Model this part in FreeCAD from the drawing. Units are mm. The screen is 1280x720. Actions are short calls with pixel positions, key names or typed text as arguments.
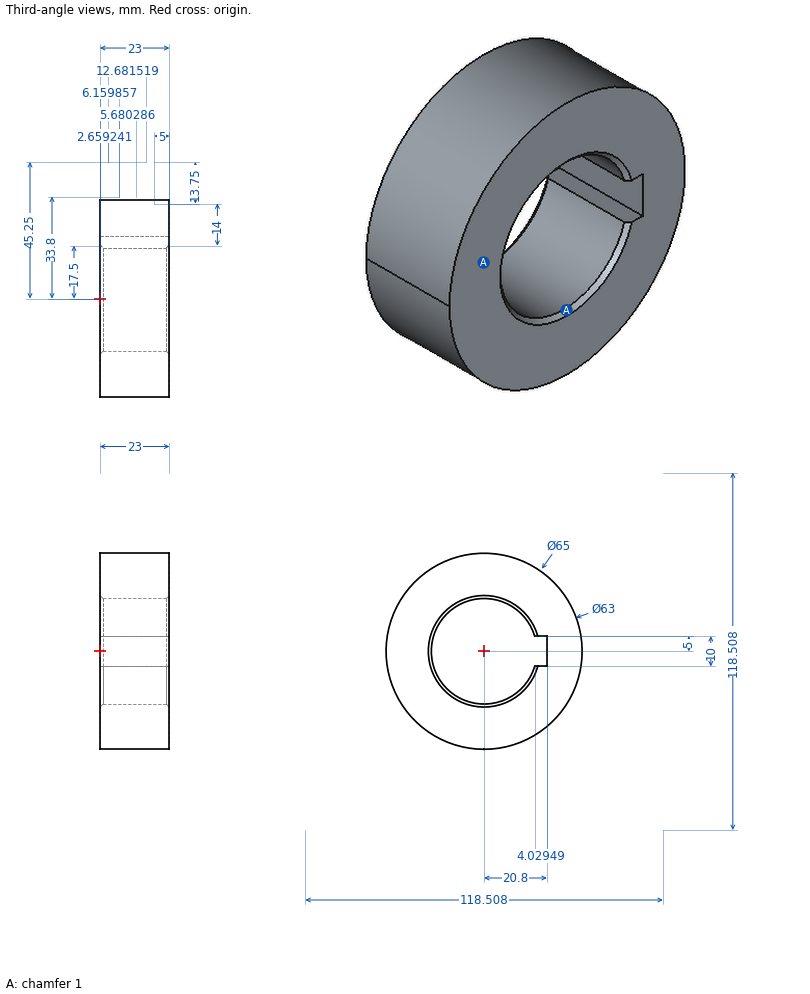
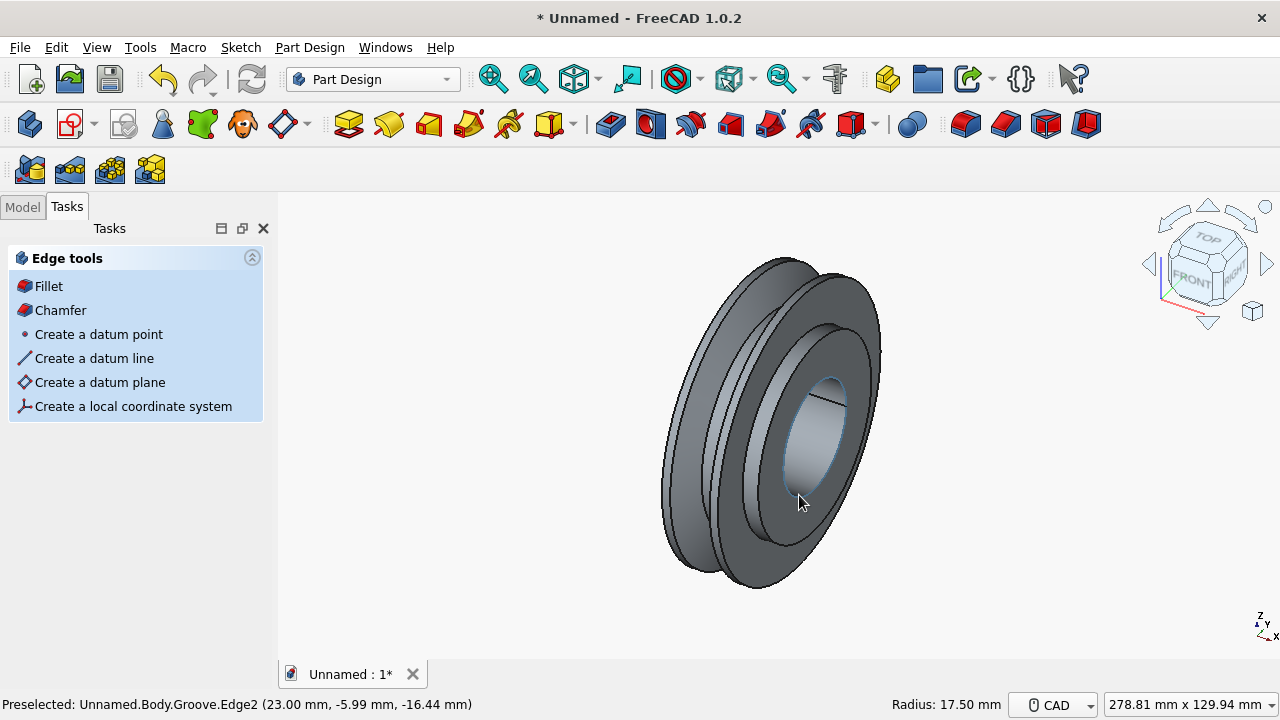
key(0)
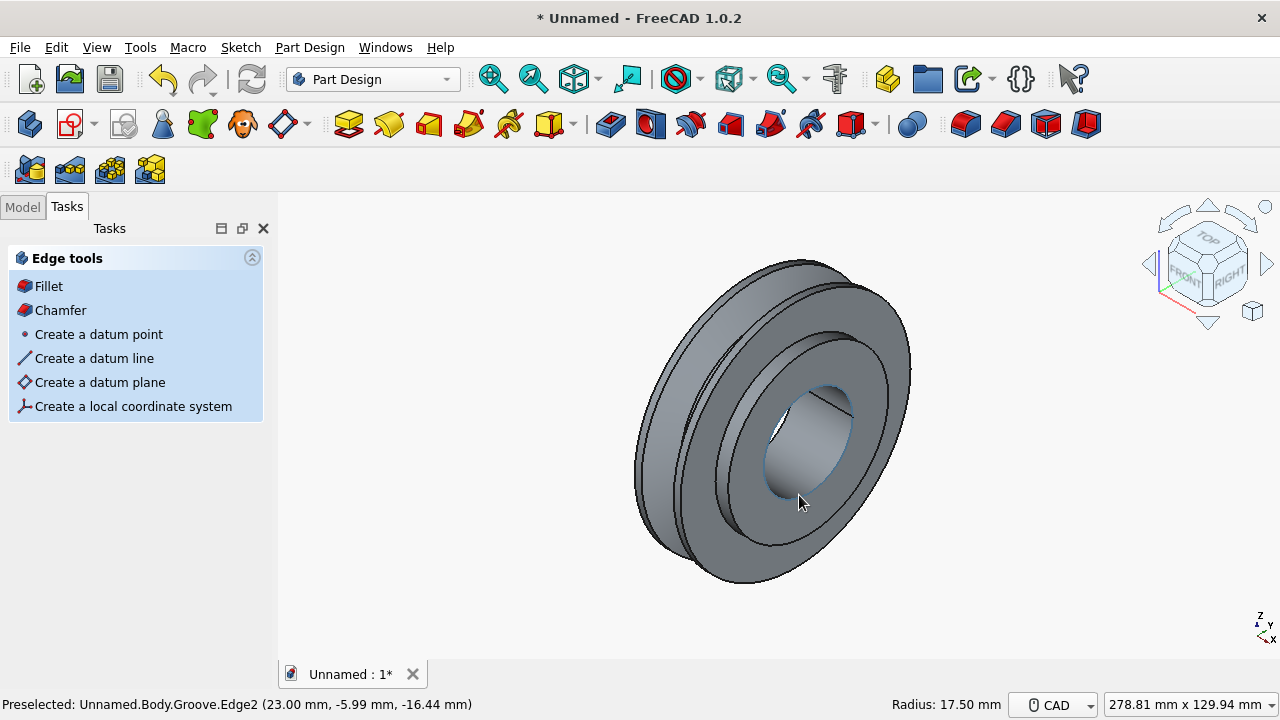
key(2)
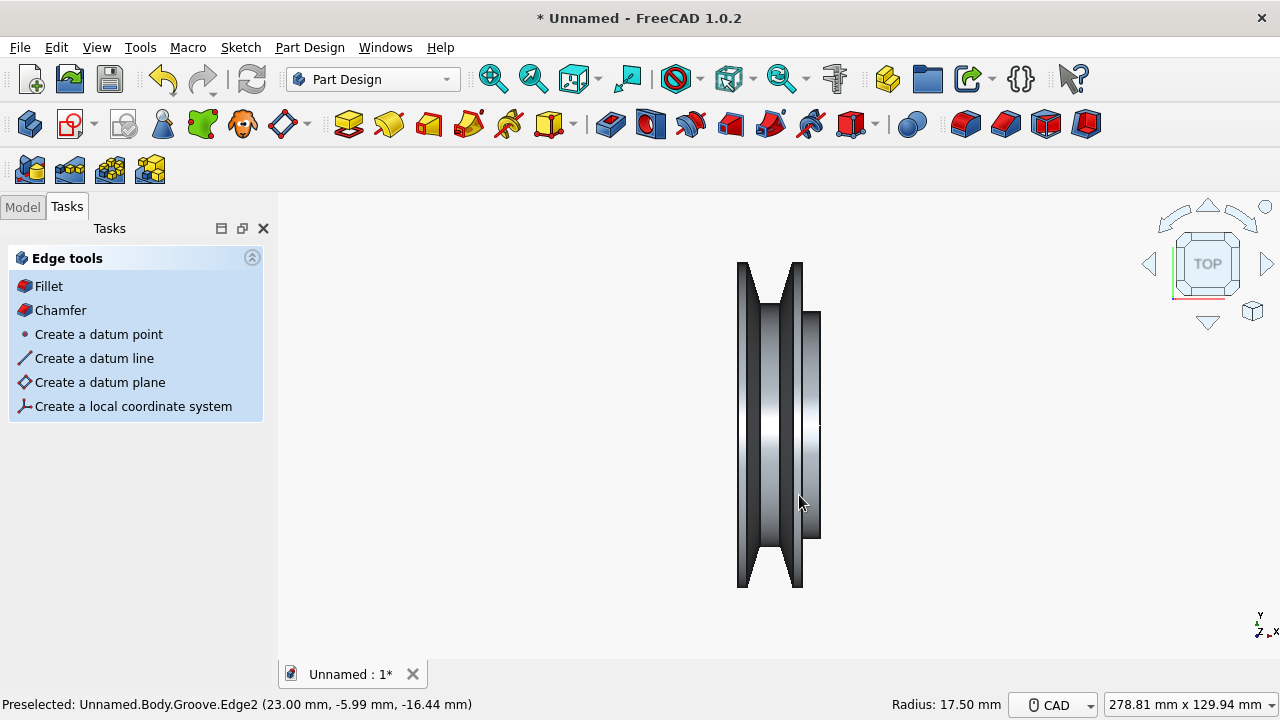
key(1)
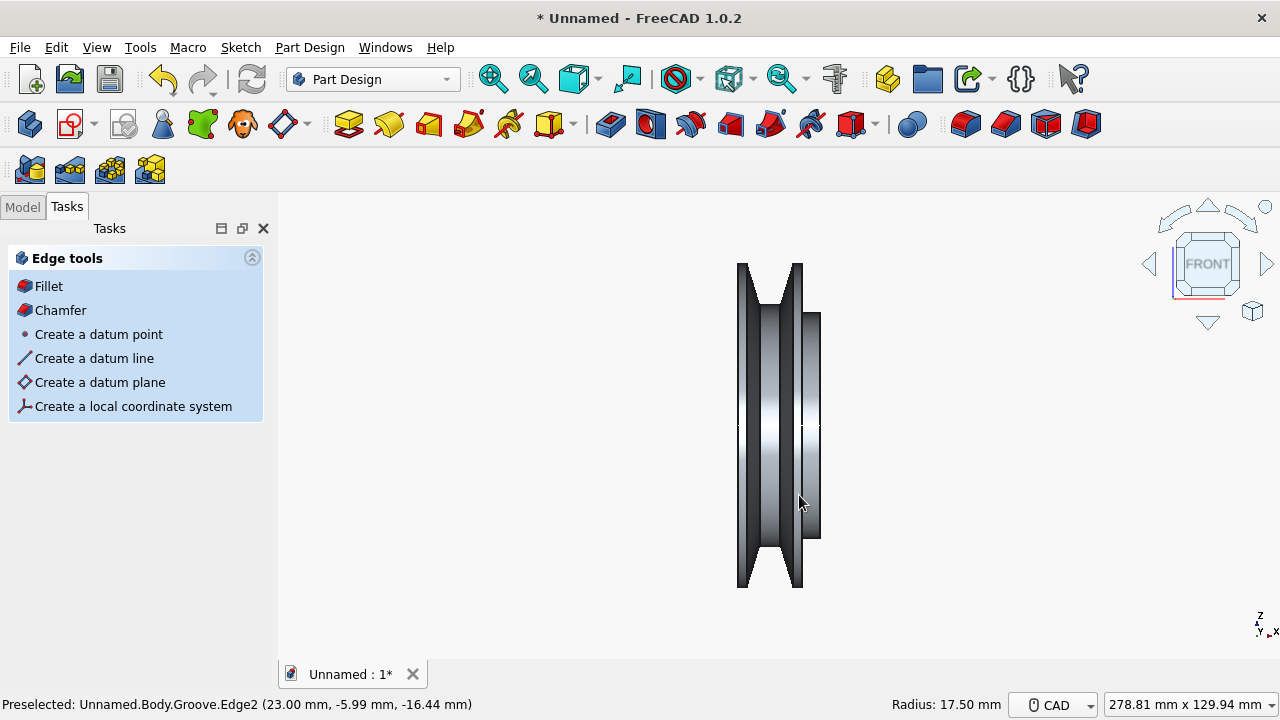
key(3)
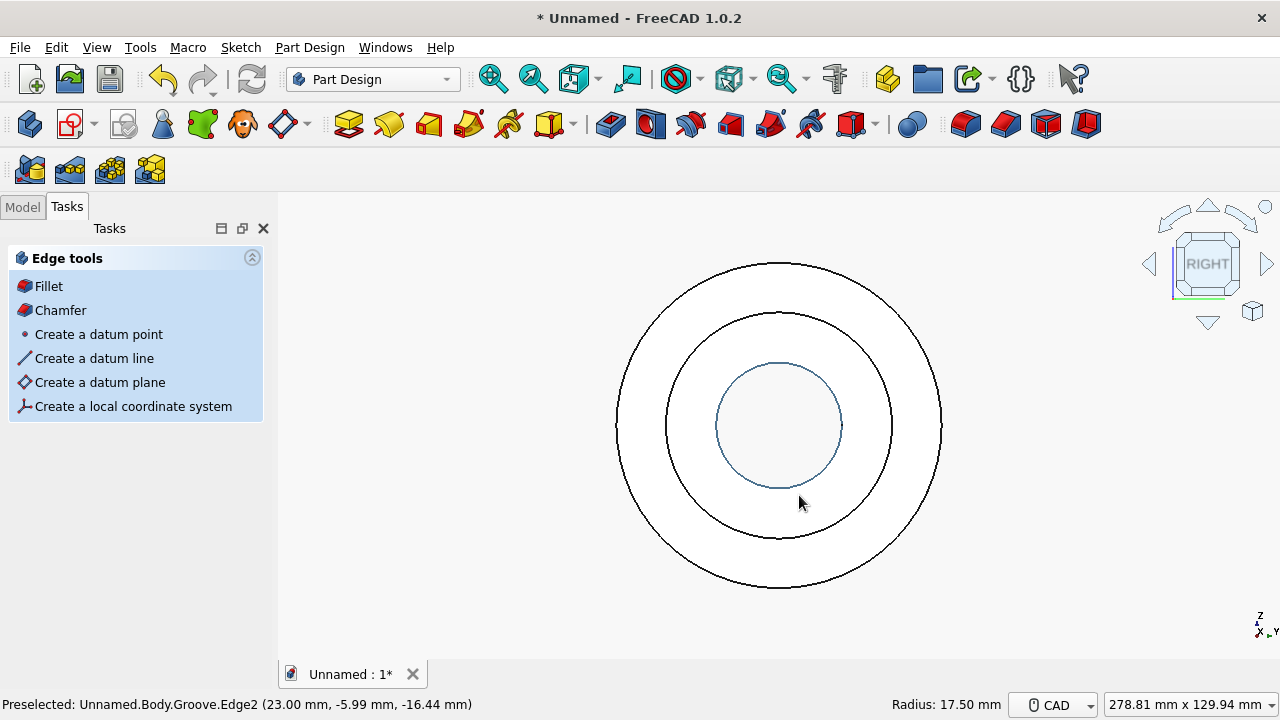
key(5)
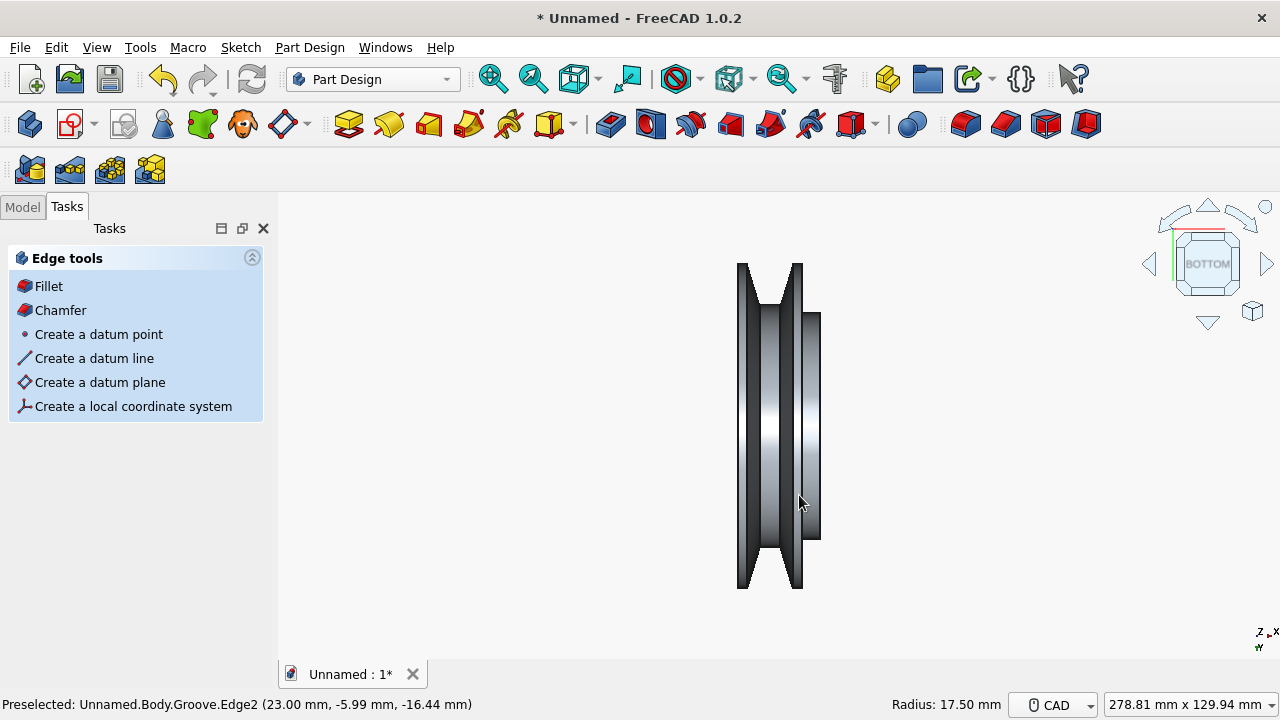
key(4)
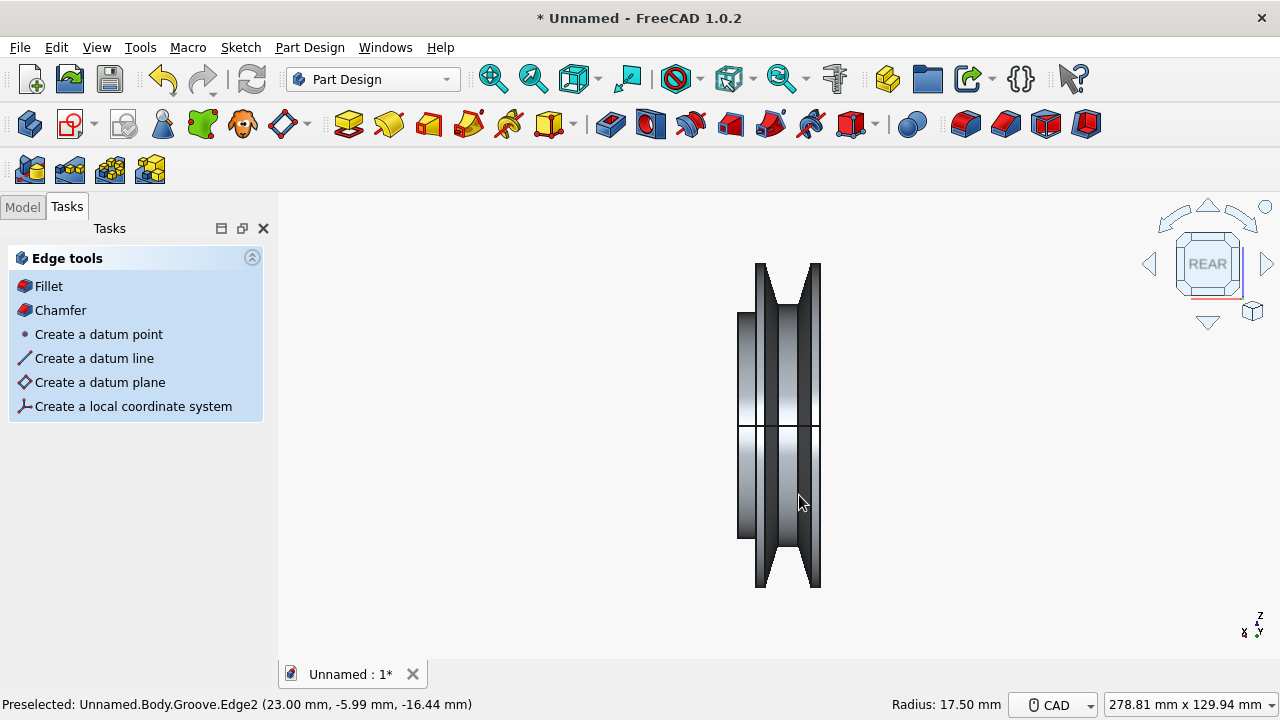
key(6)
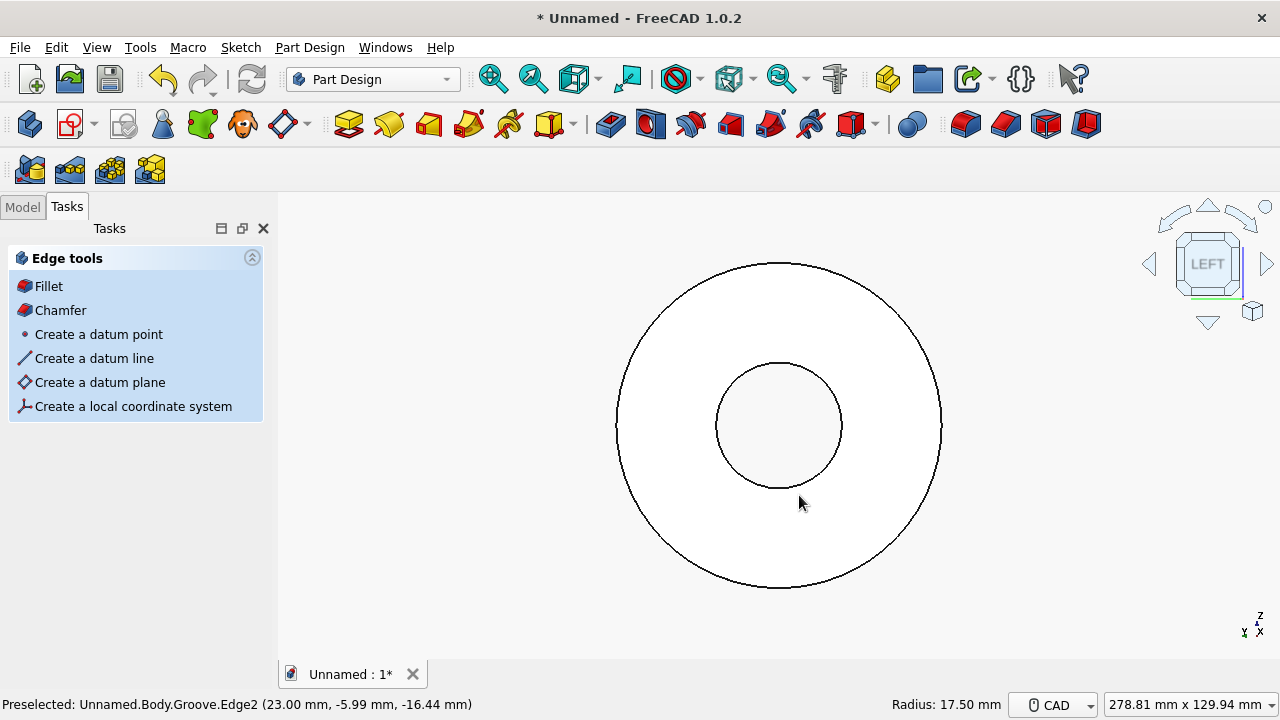
click(842, 424, ctrl)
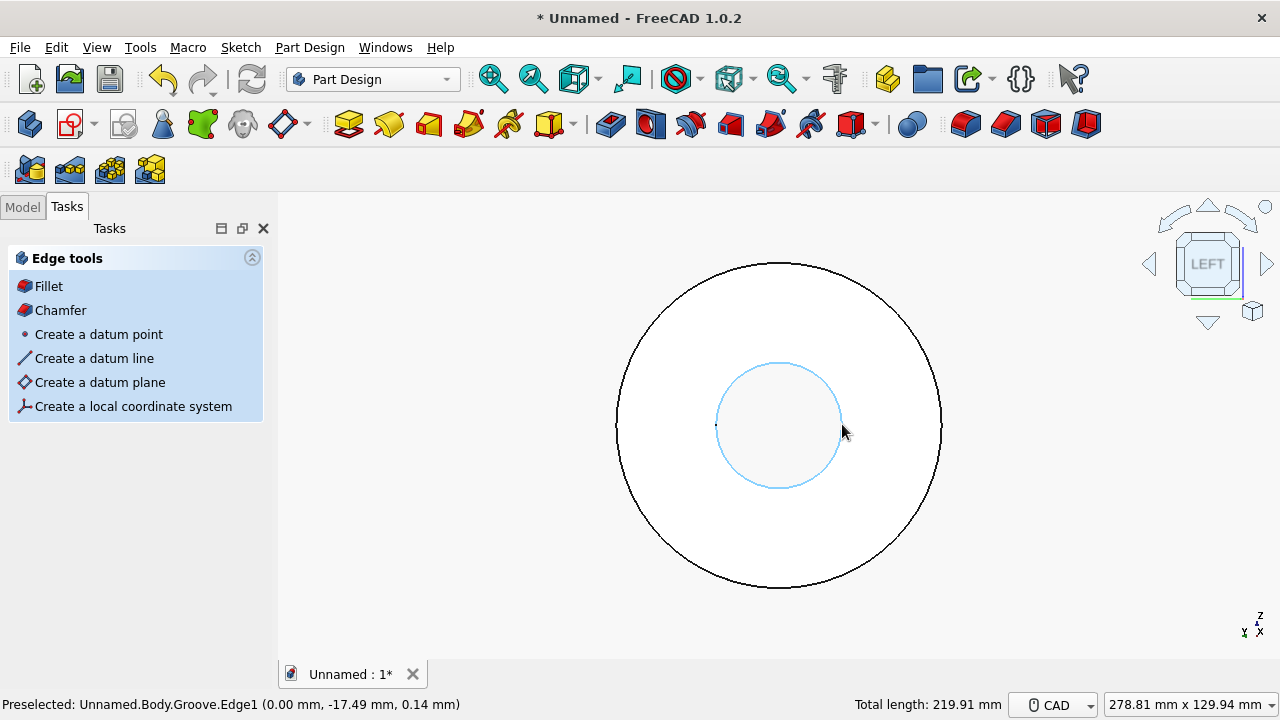
click(1006, 124)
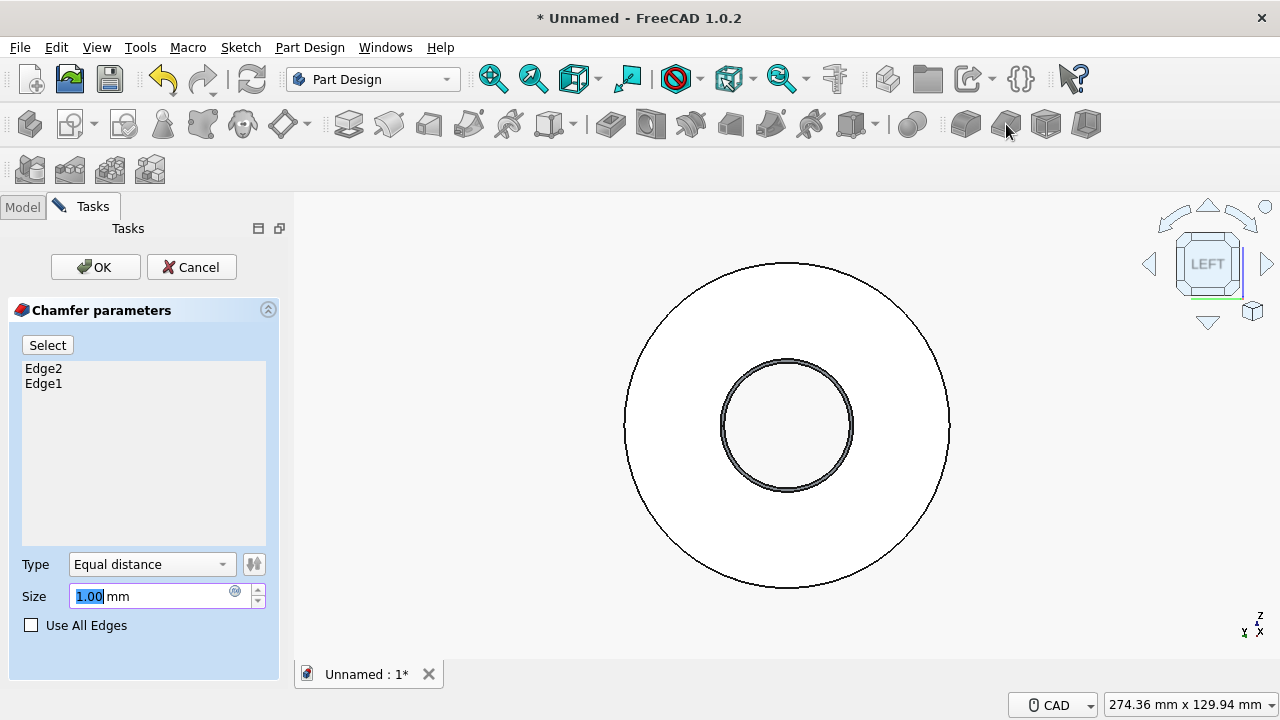
text(1)
key(Tab)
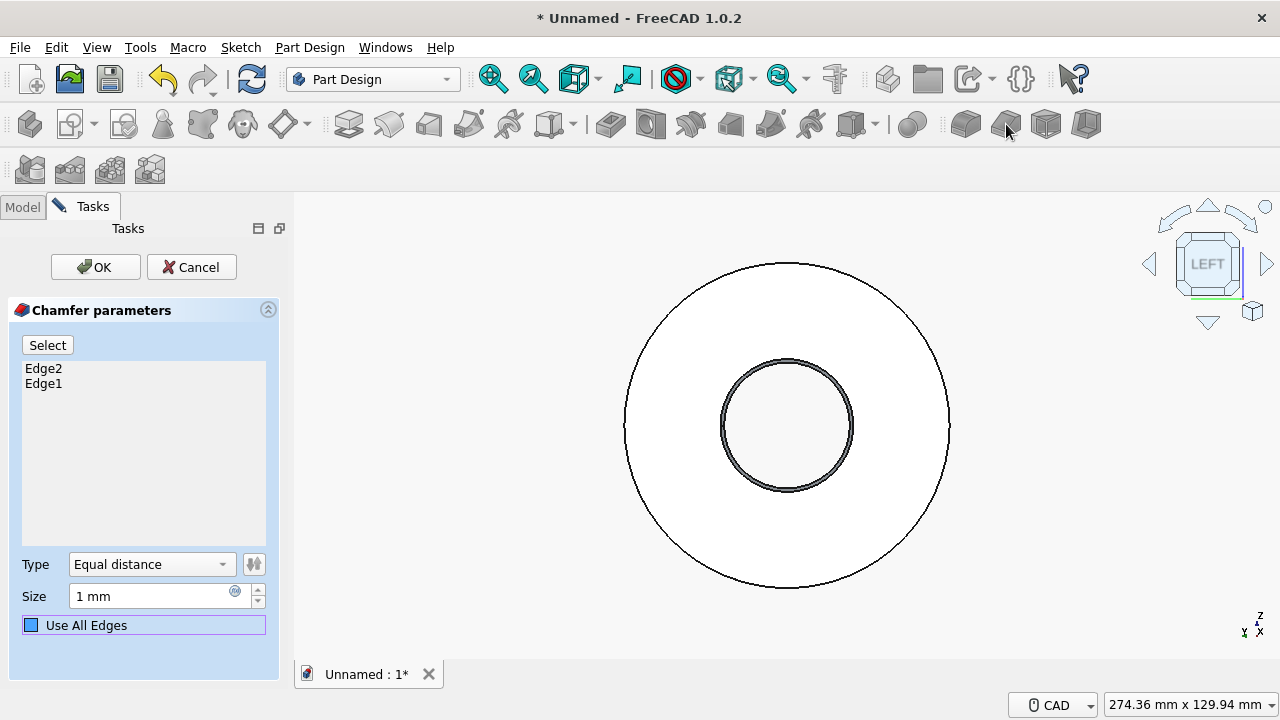
click(96, 267)